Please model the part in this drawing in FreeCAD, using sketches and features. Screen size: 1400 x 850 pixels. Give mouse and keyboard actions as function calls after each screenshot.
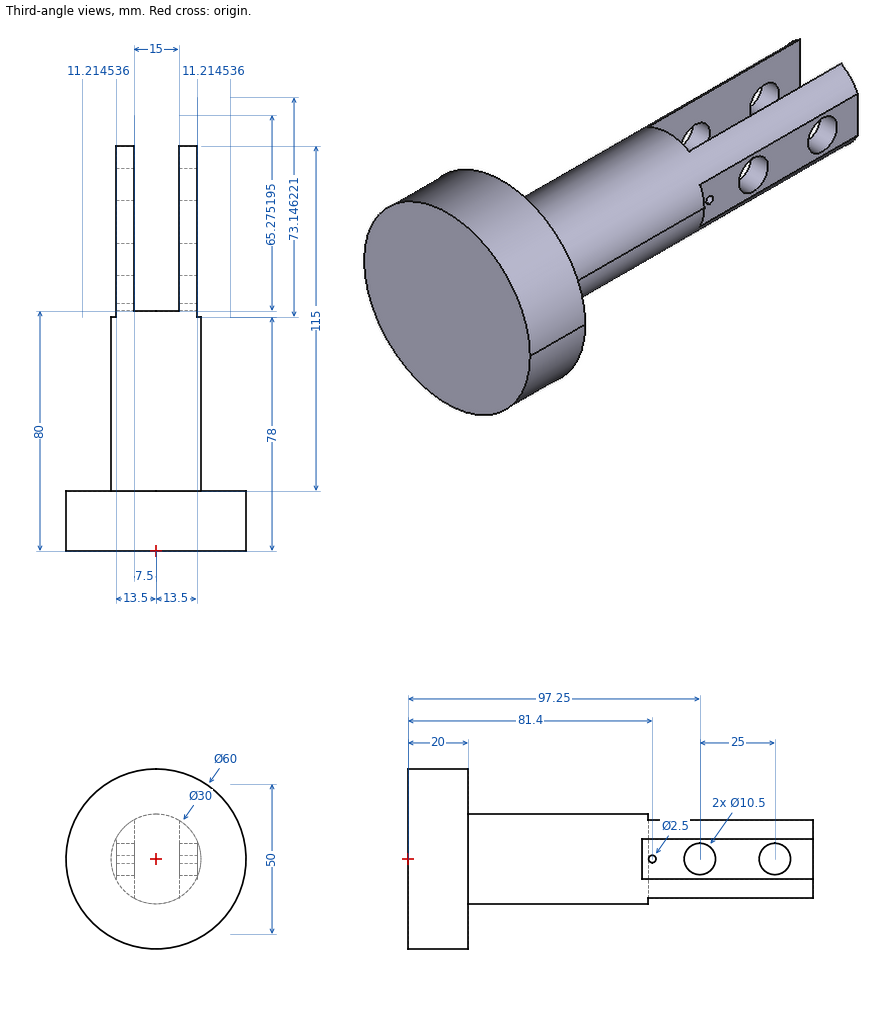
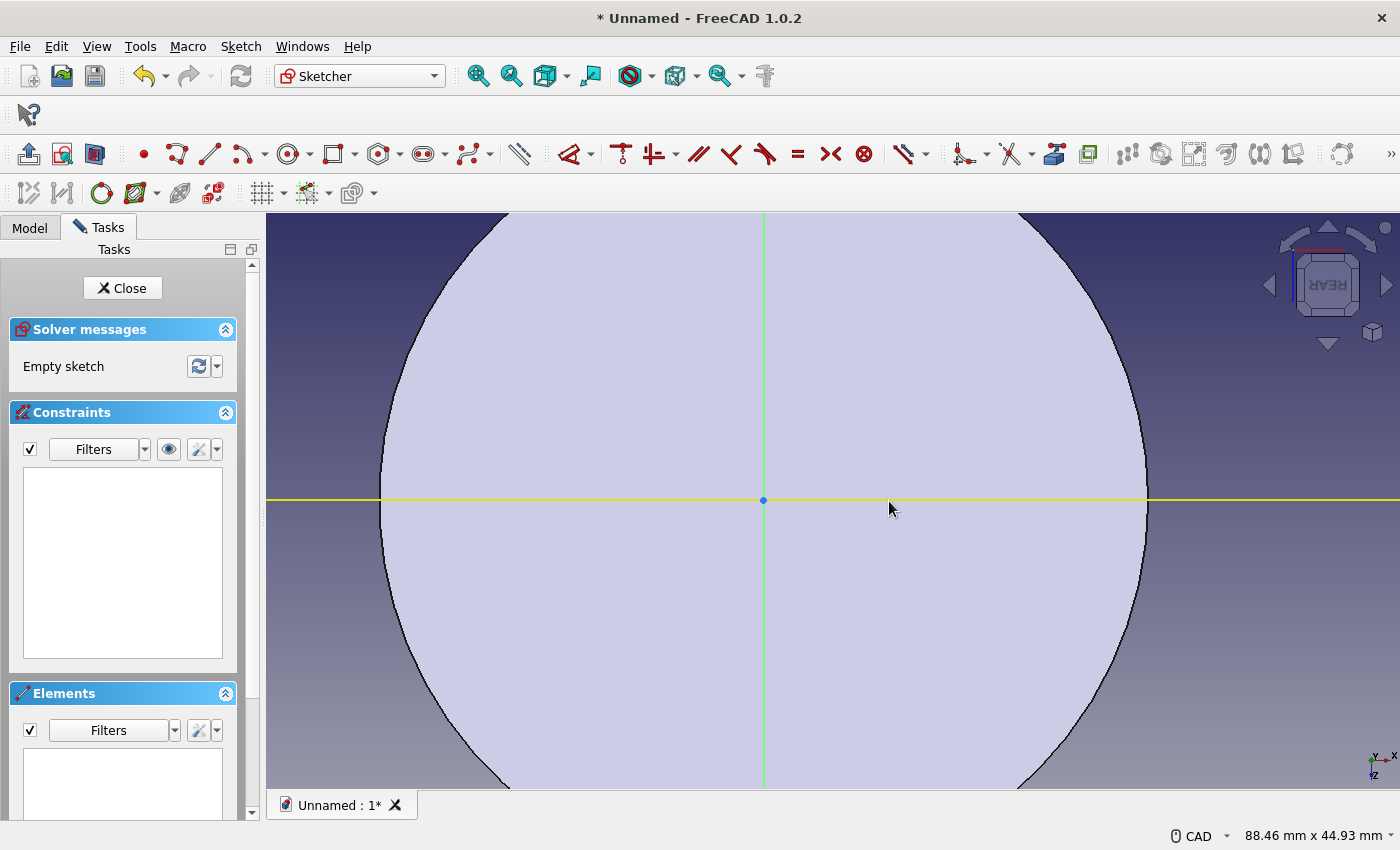
click(288, 154)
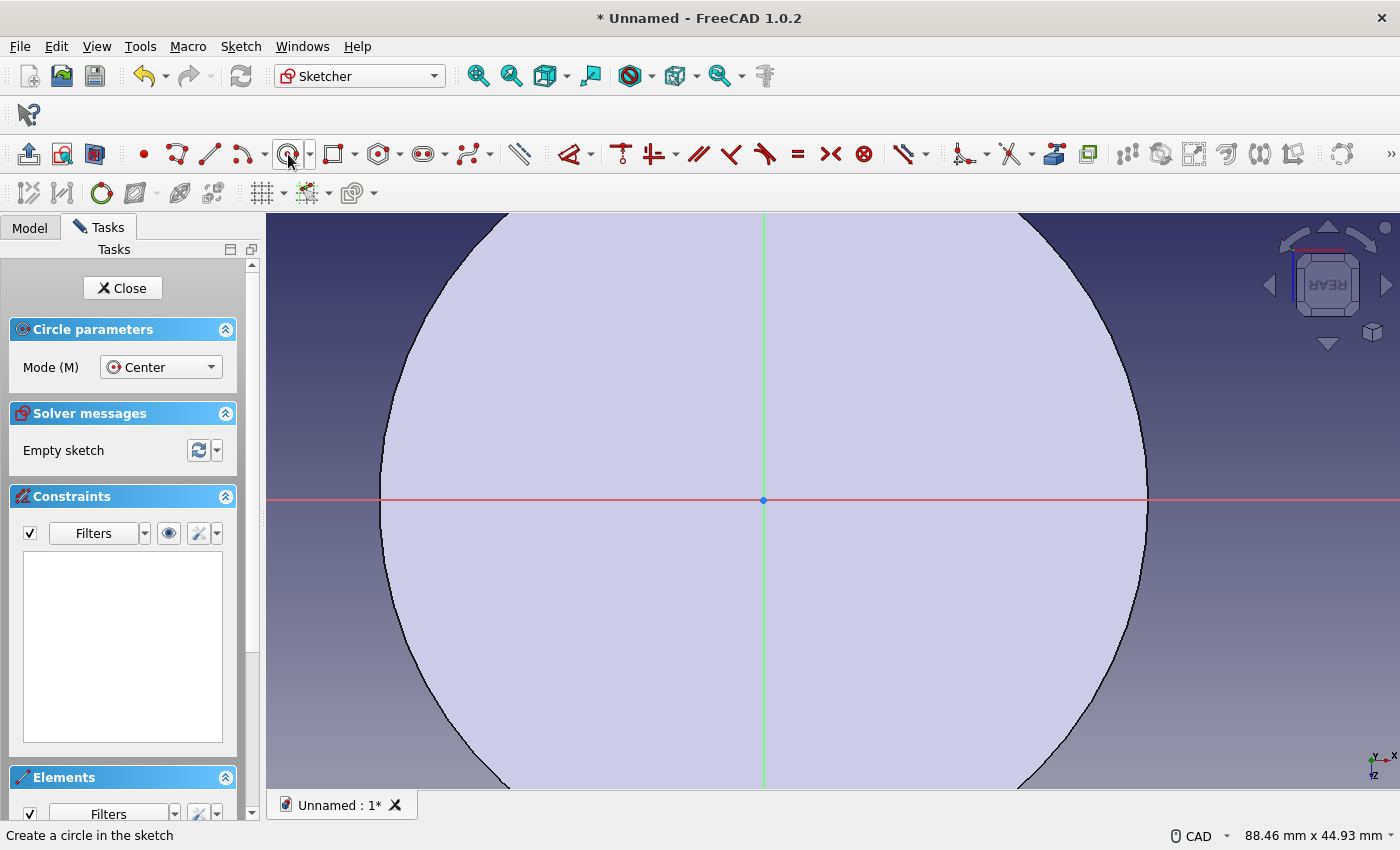
click(764, 500)
move(900, 364)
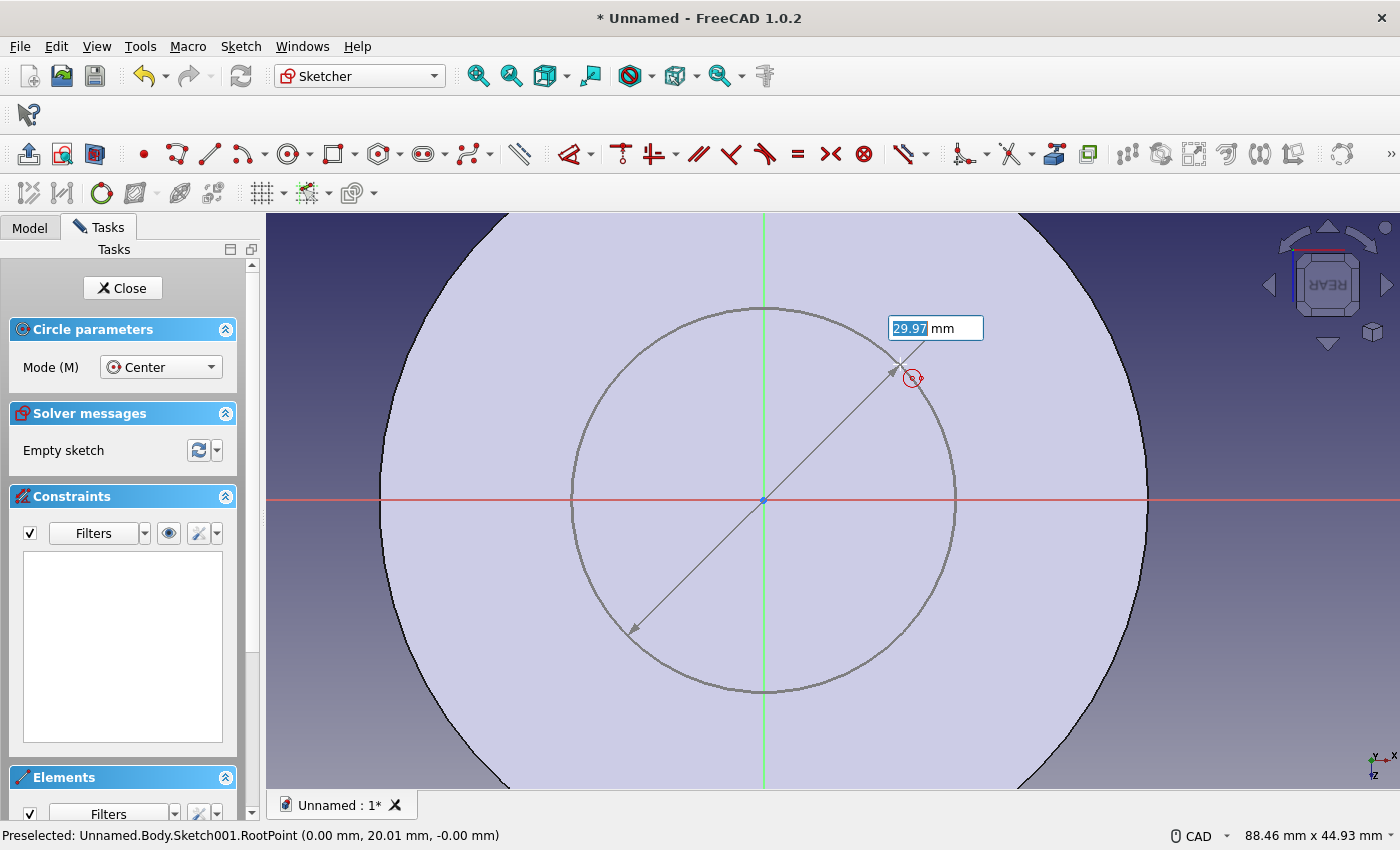
text(30)
key(Return)
key(Escape)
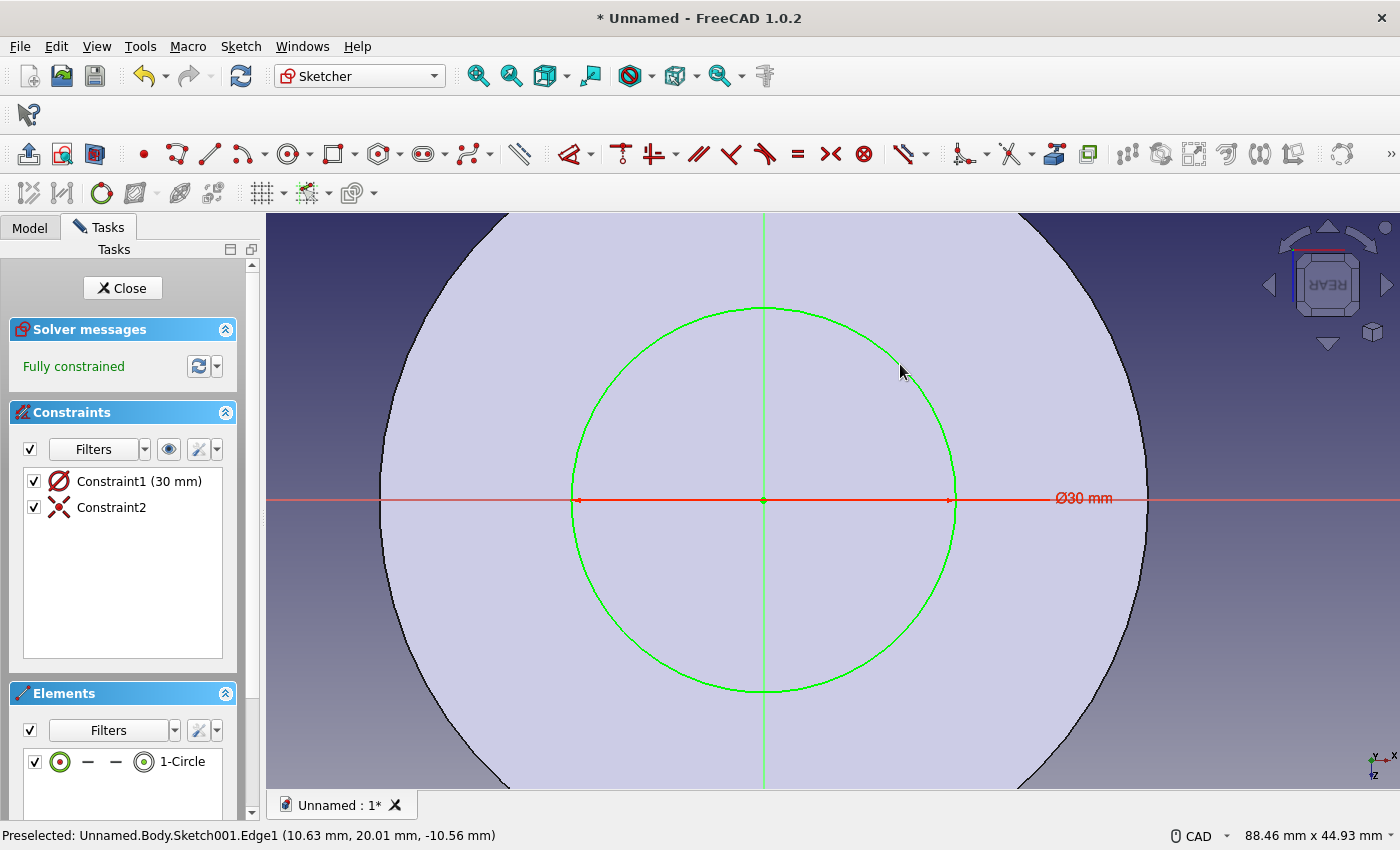
click(123, 288)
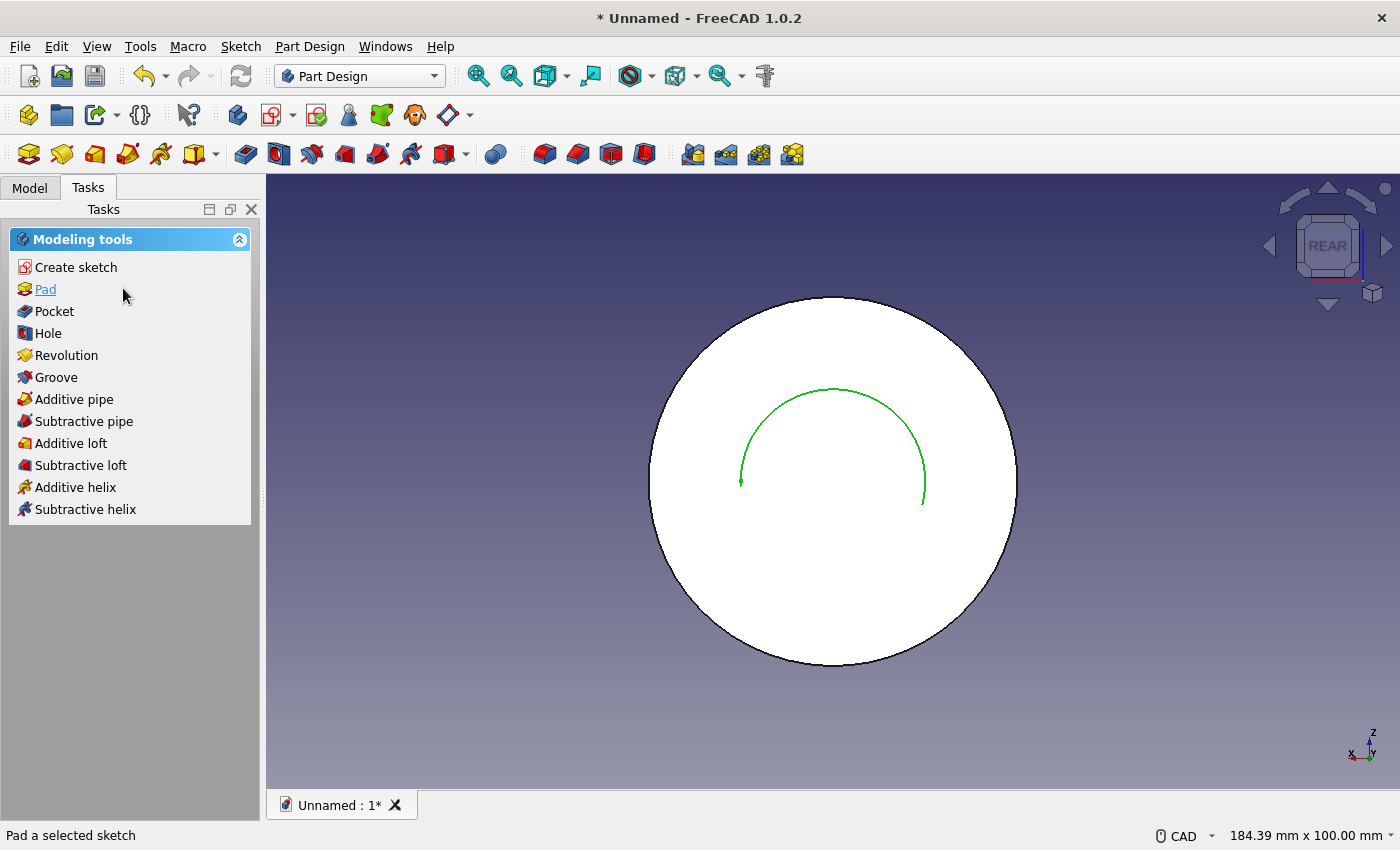
click(29, 154)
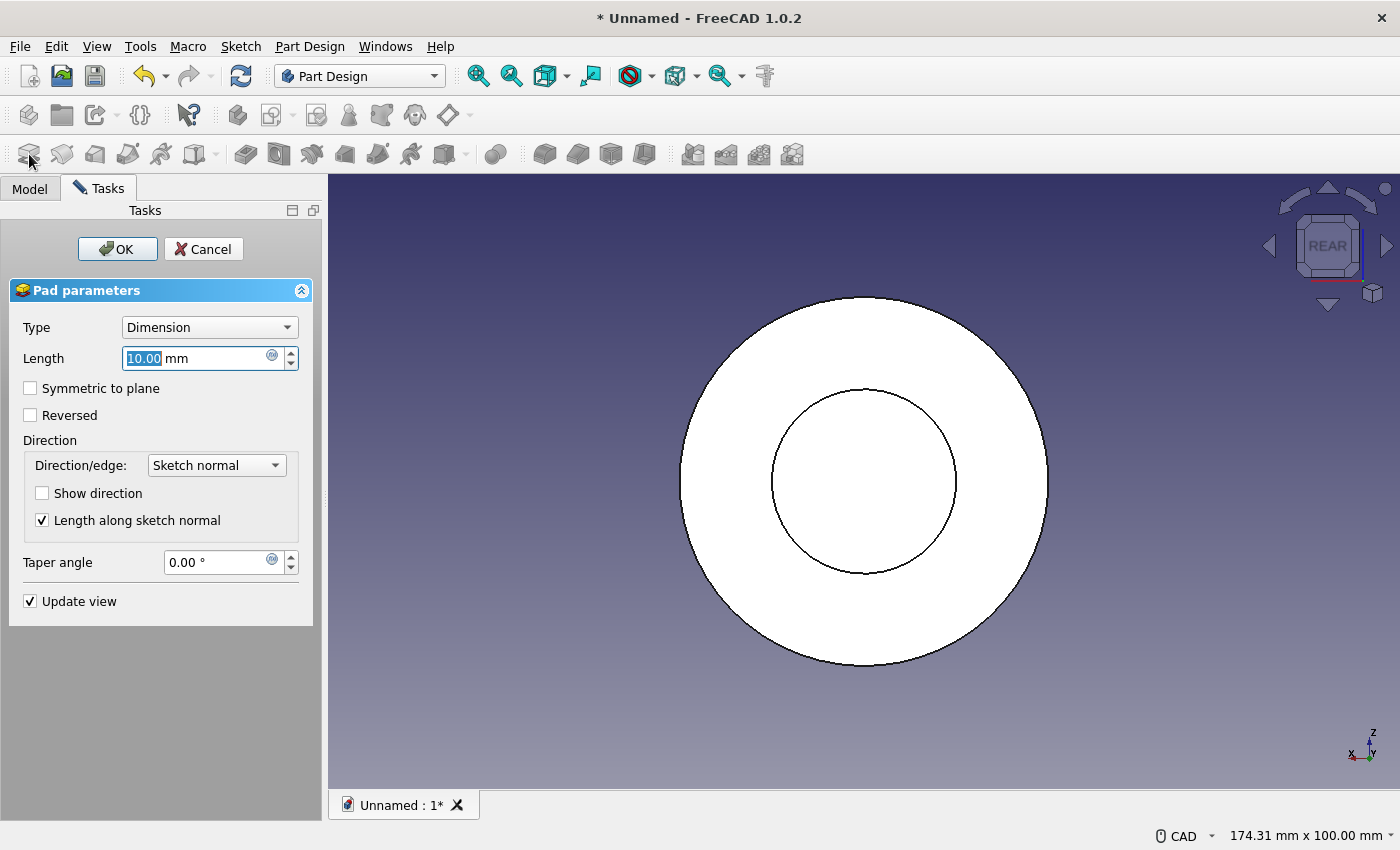
text(115)
key(Tab)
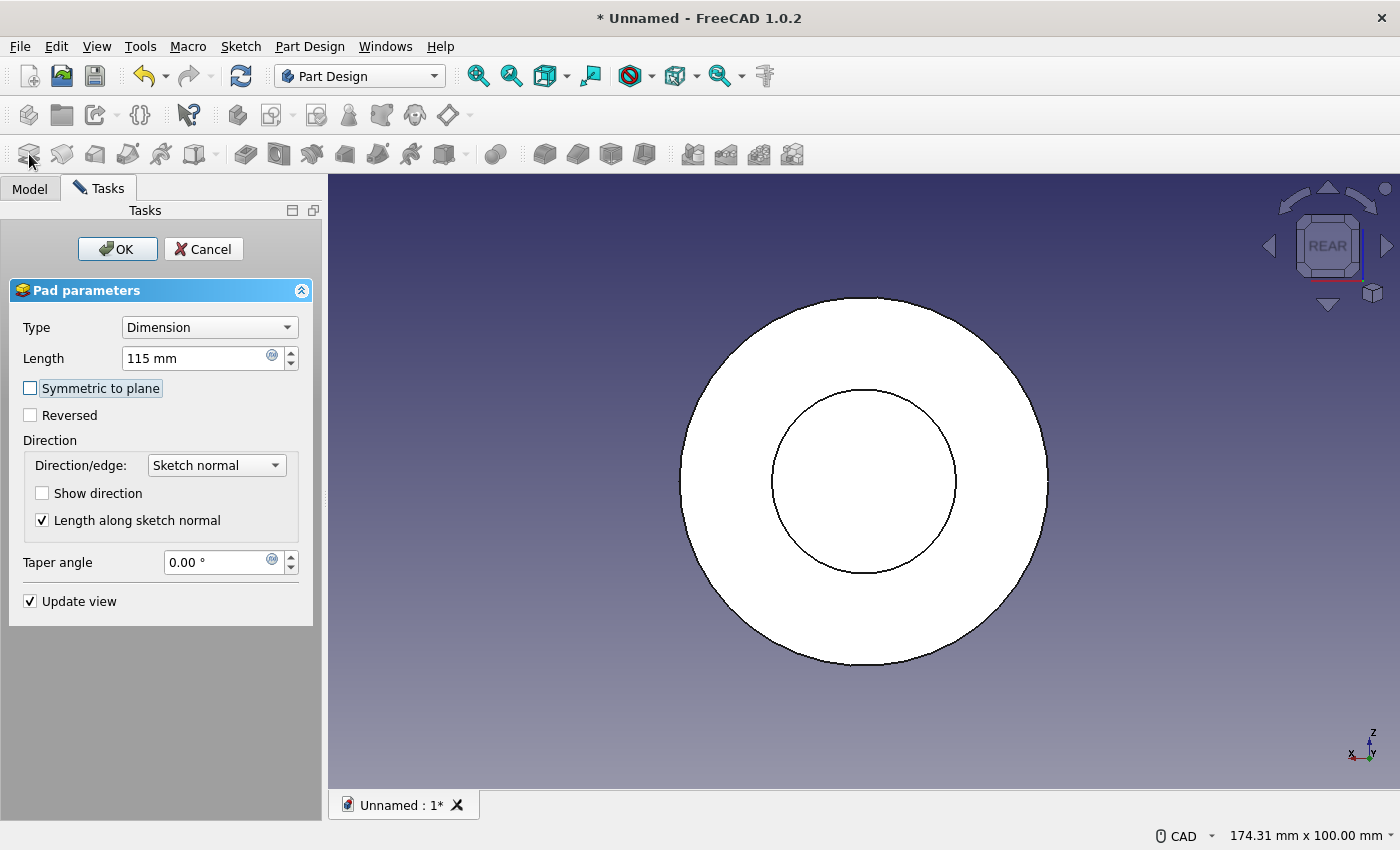
click(118, 249)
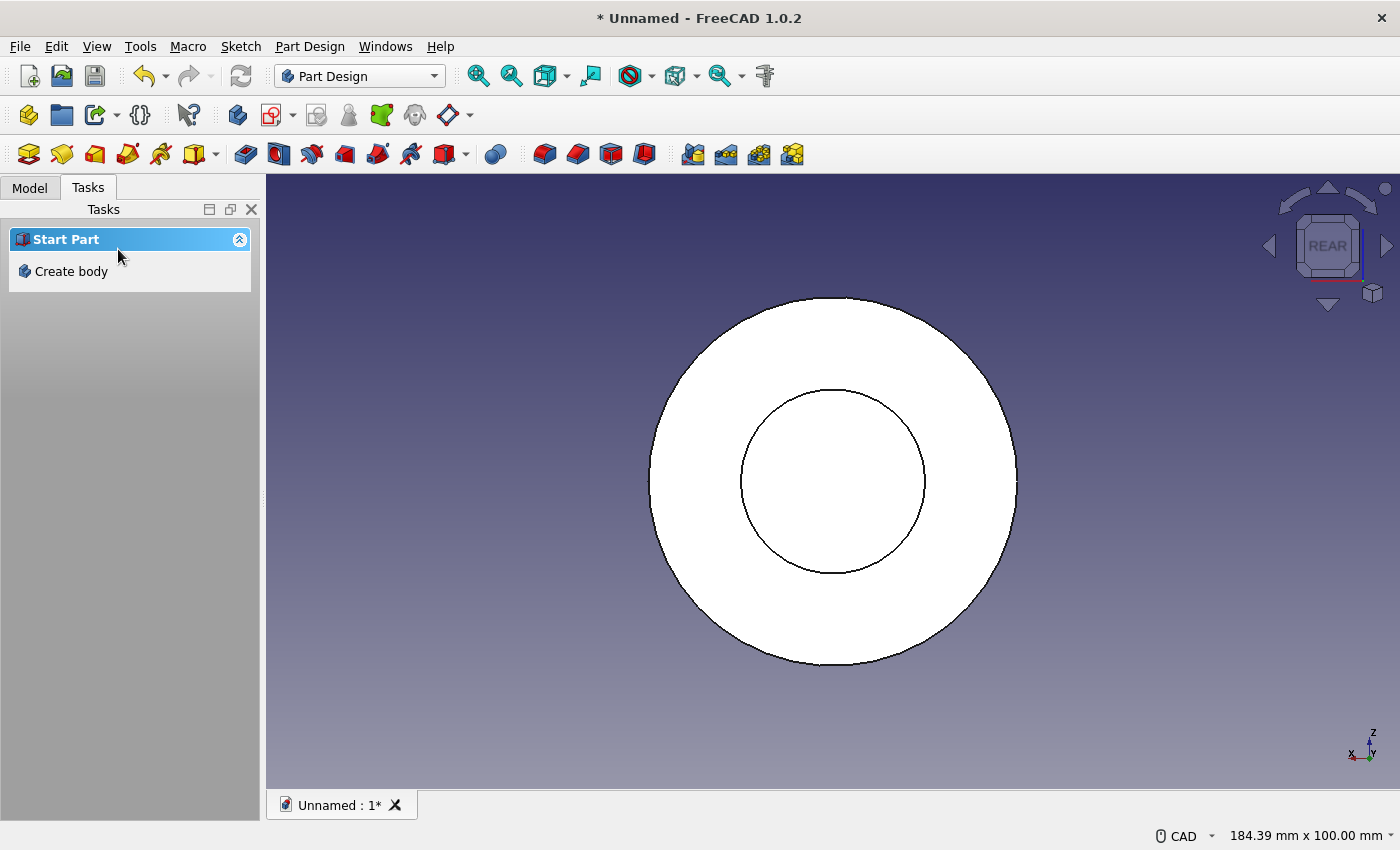
click(270, 116)